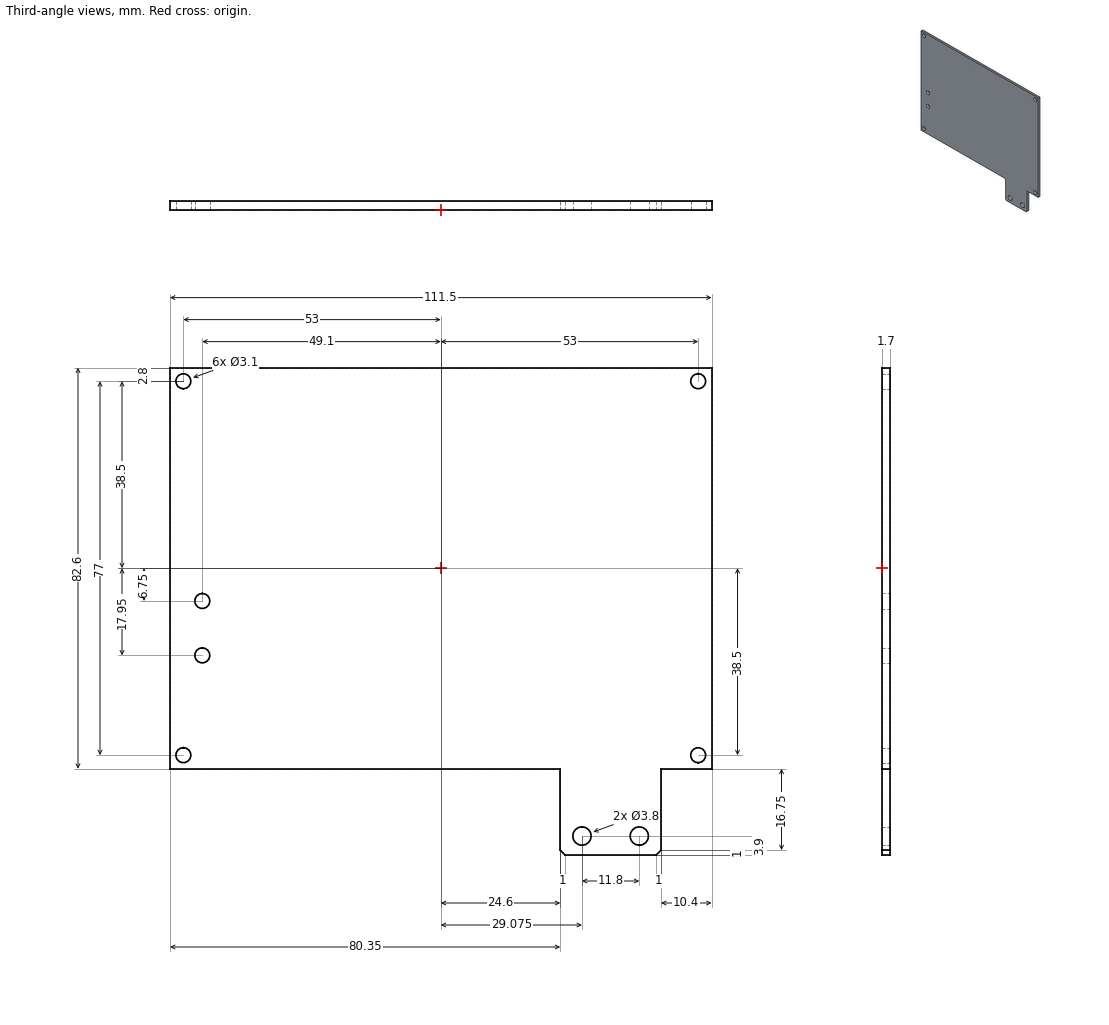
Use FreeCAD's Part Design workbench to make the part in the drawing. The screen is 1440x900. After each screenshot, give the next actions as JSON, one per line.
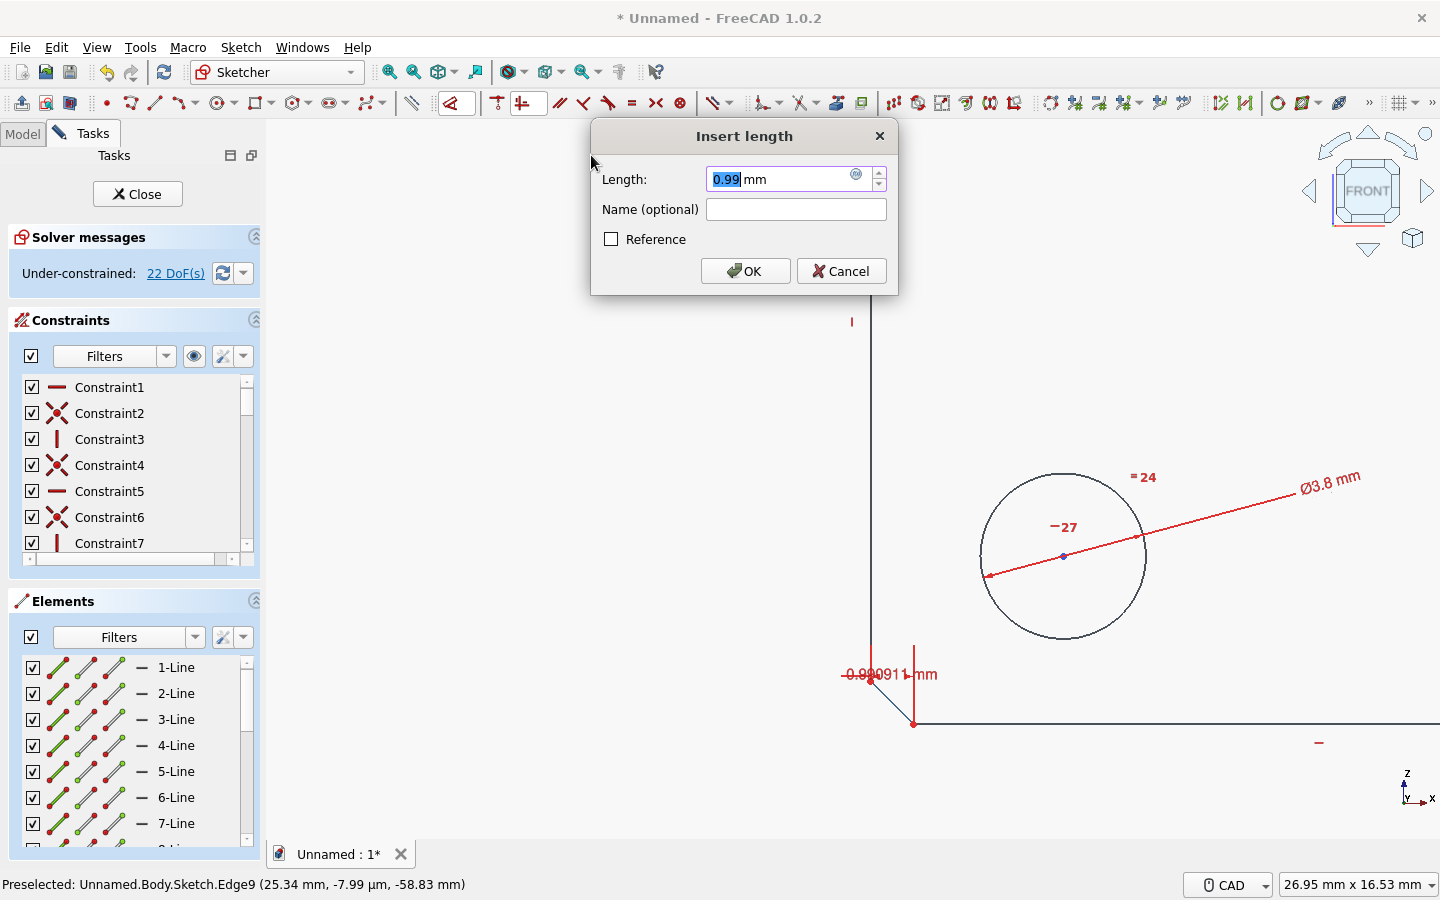
{"action": "type", "text": "1"}
{"action": "key", "text": "Return"}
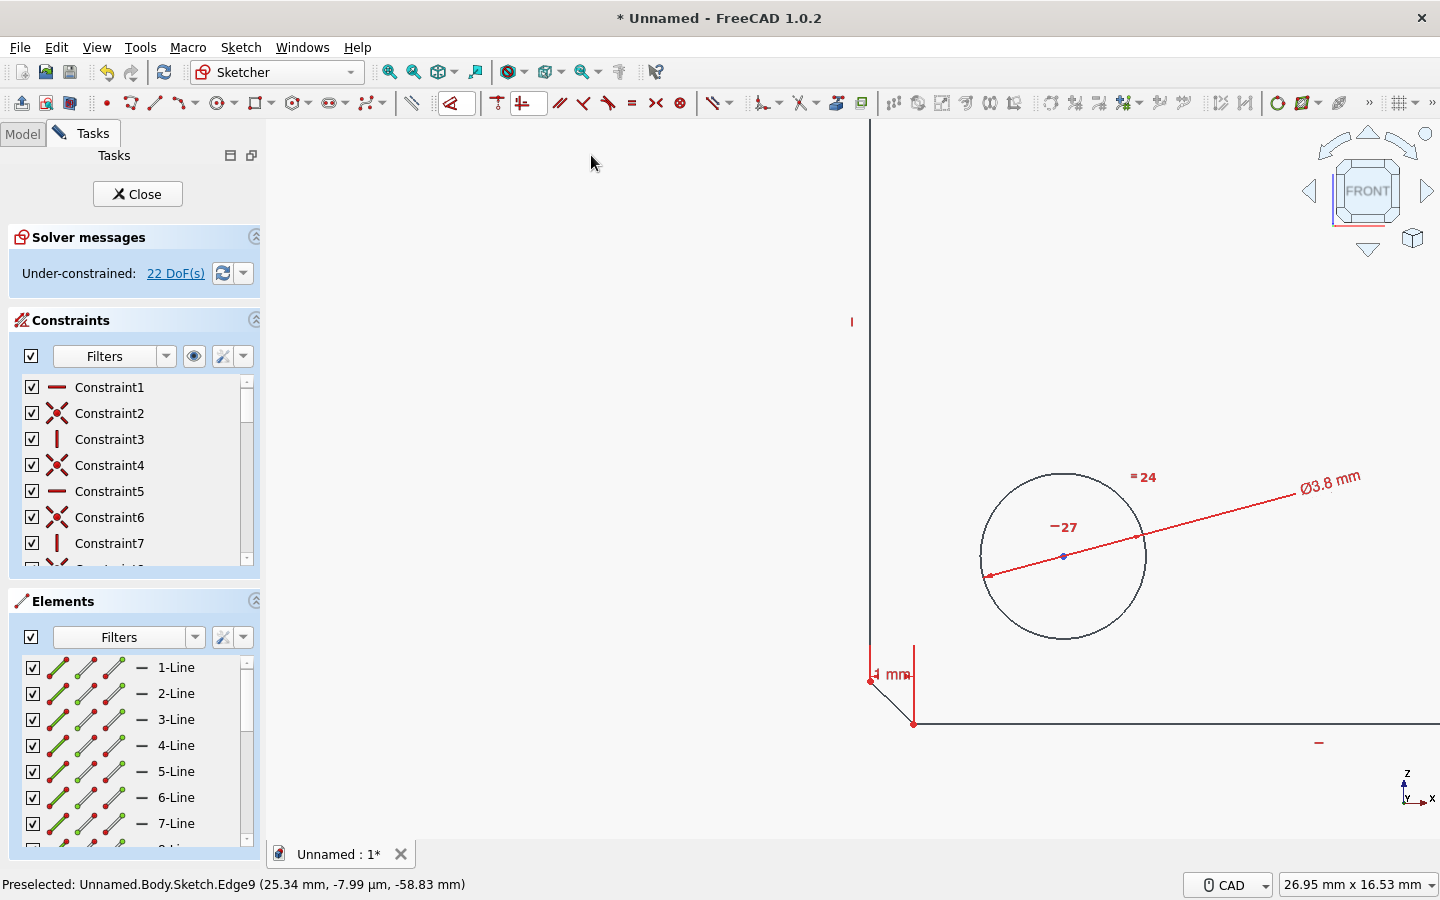
{"action": "left_click", "coordinate": [901, 712]}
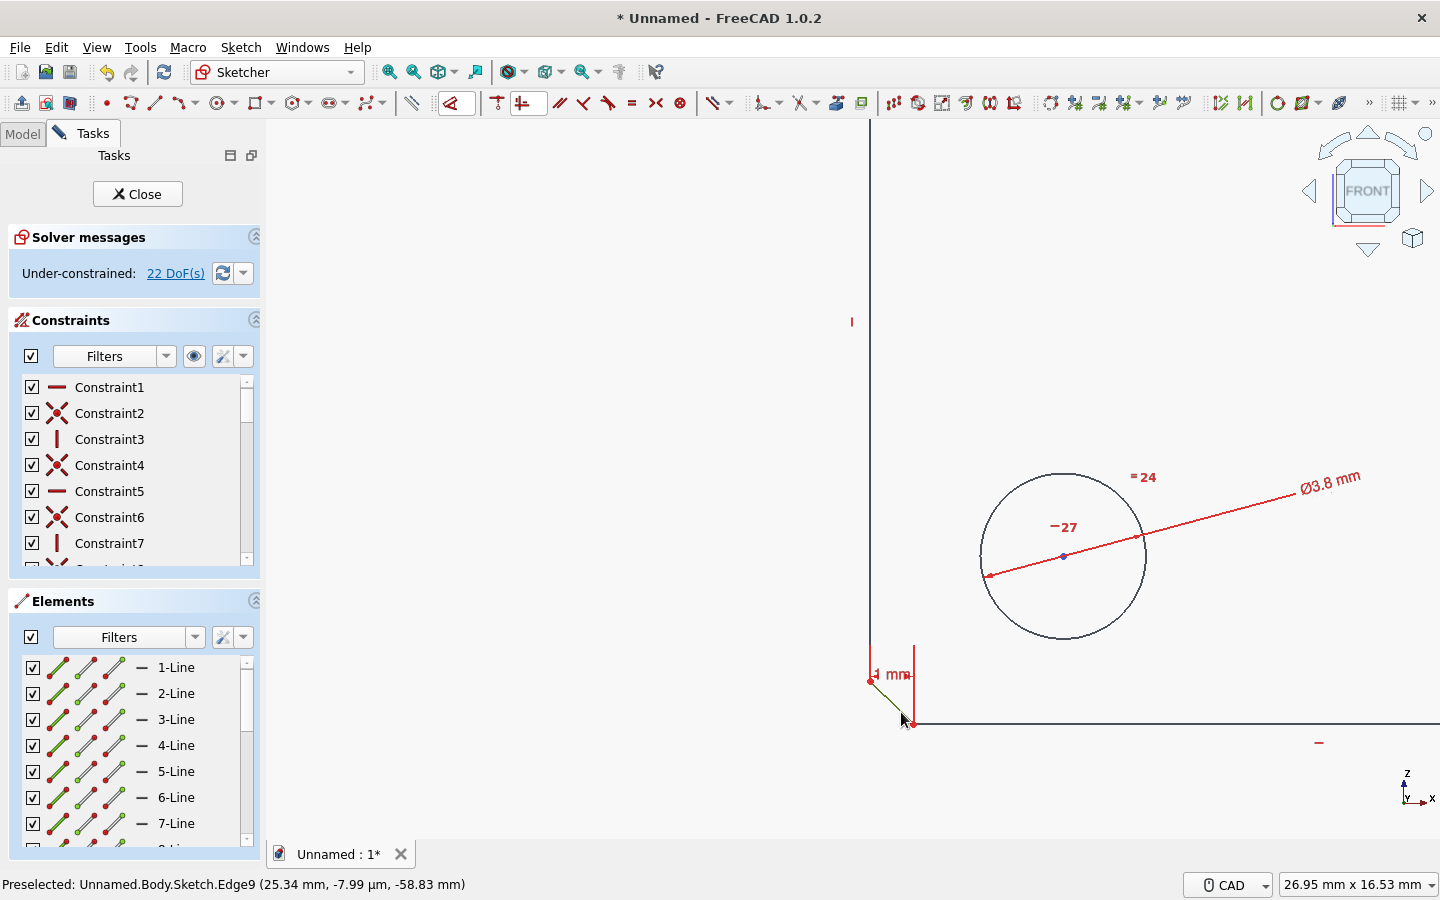
{"action": "left_click", "coordinate": [470, 104]}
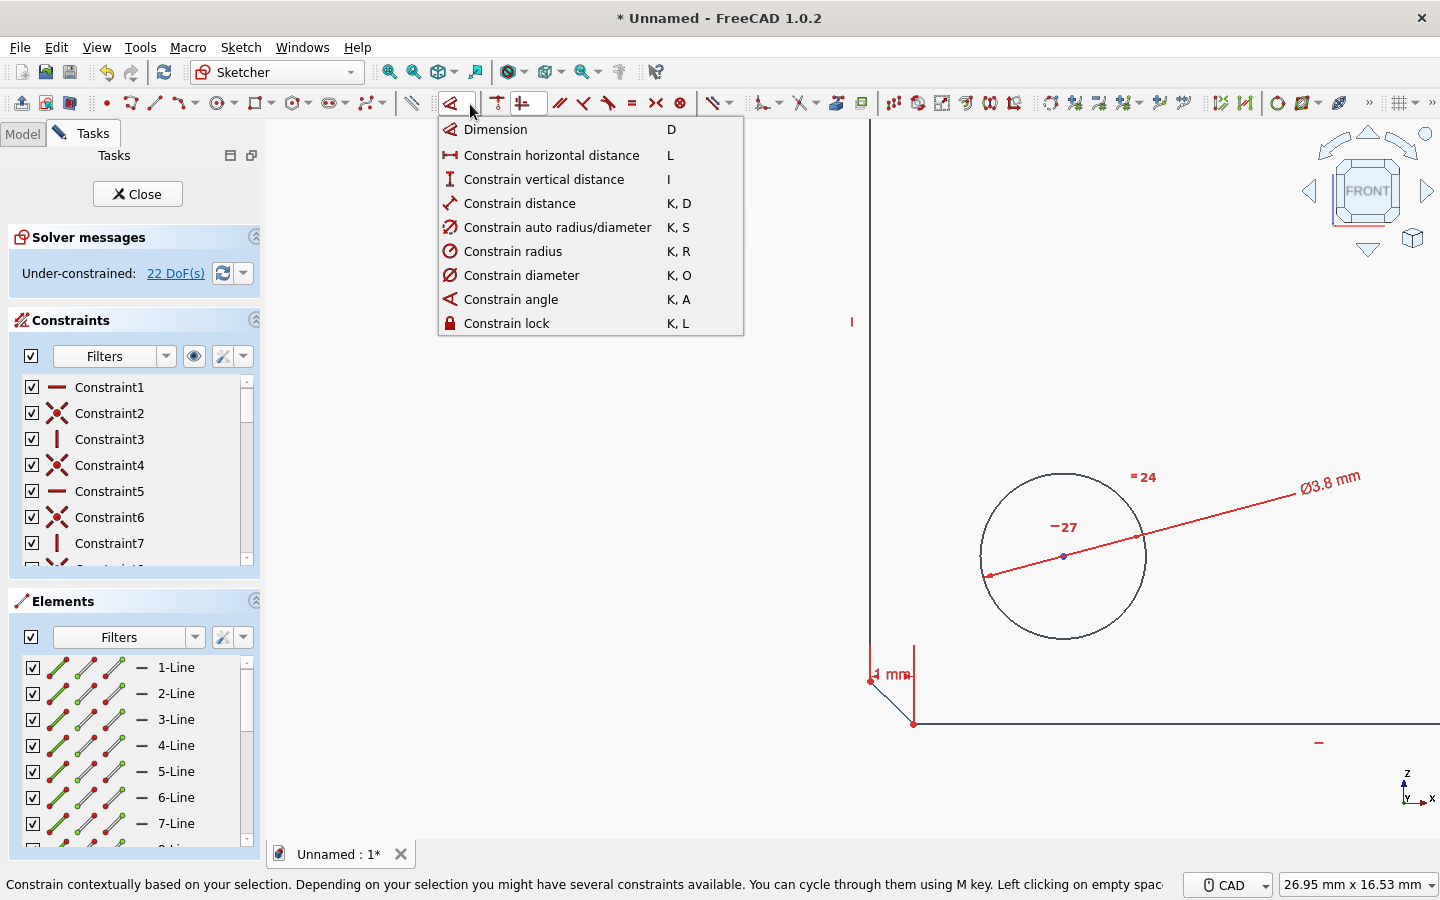
{"action": "left_click", "coordinate": [591, 179]}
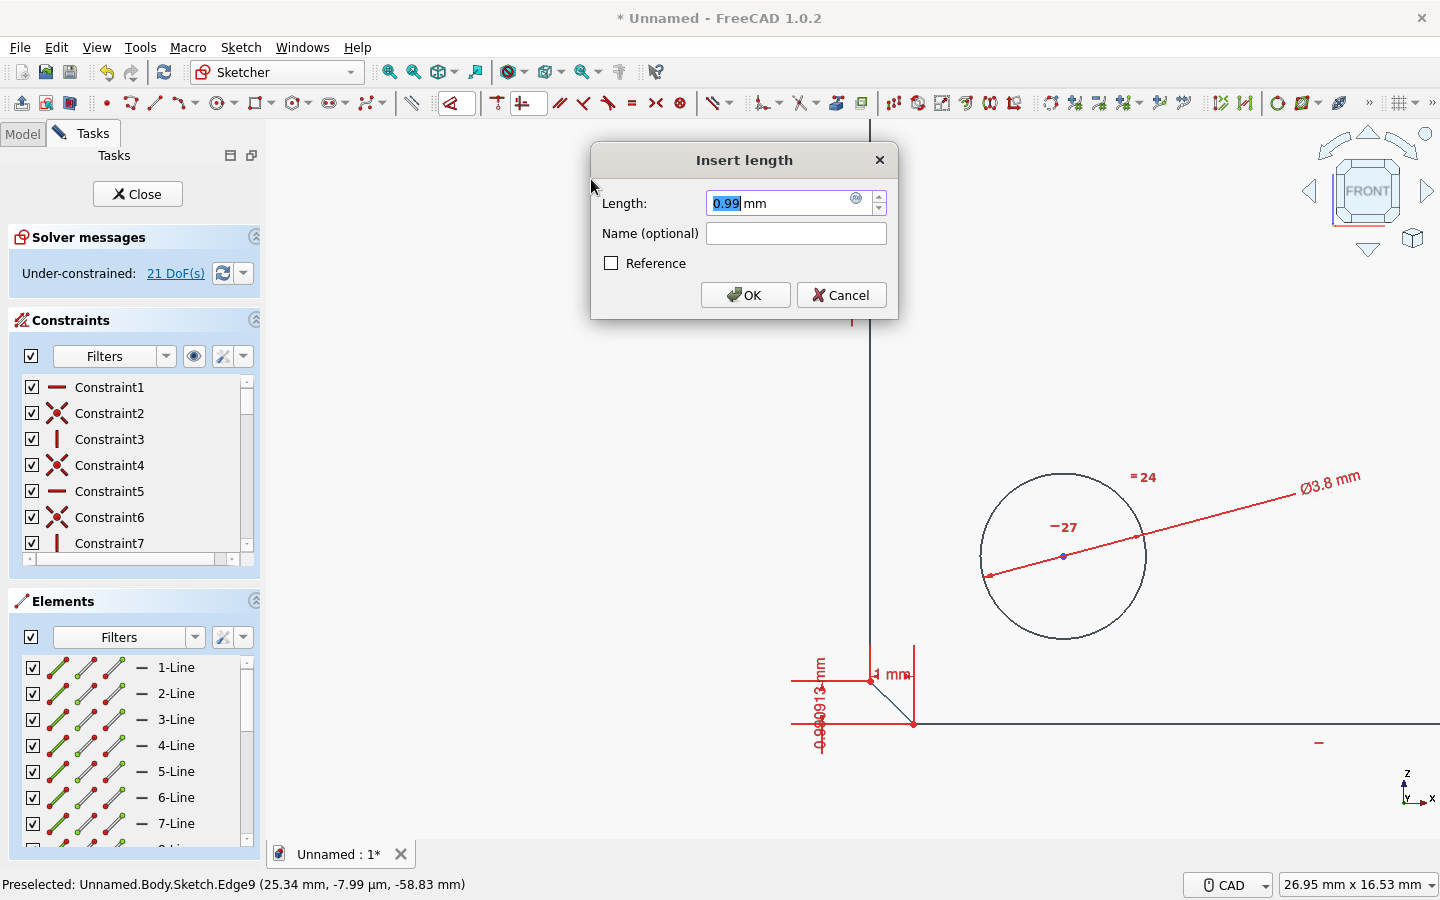
{"action": "type", "text": "1"}
{"action": "key", "text": "Return"}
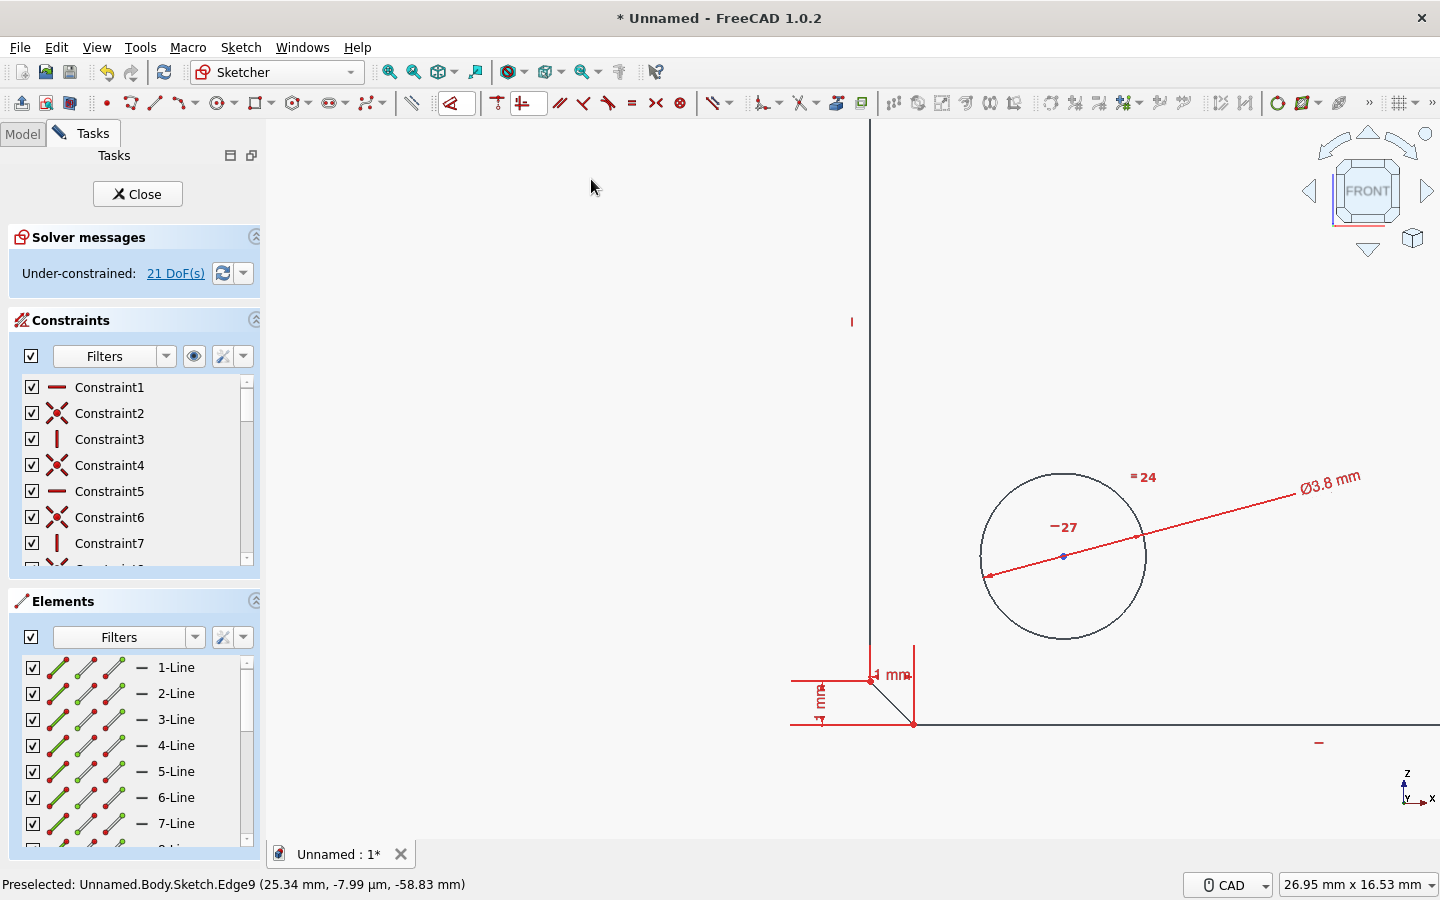
{"action": "scroll", "coordinate": [907, 721], "scroll_direction": "down", "scroll_amount": 11}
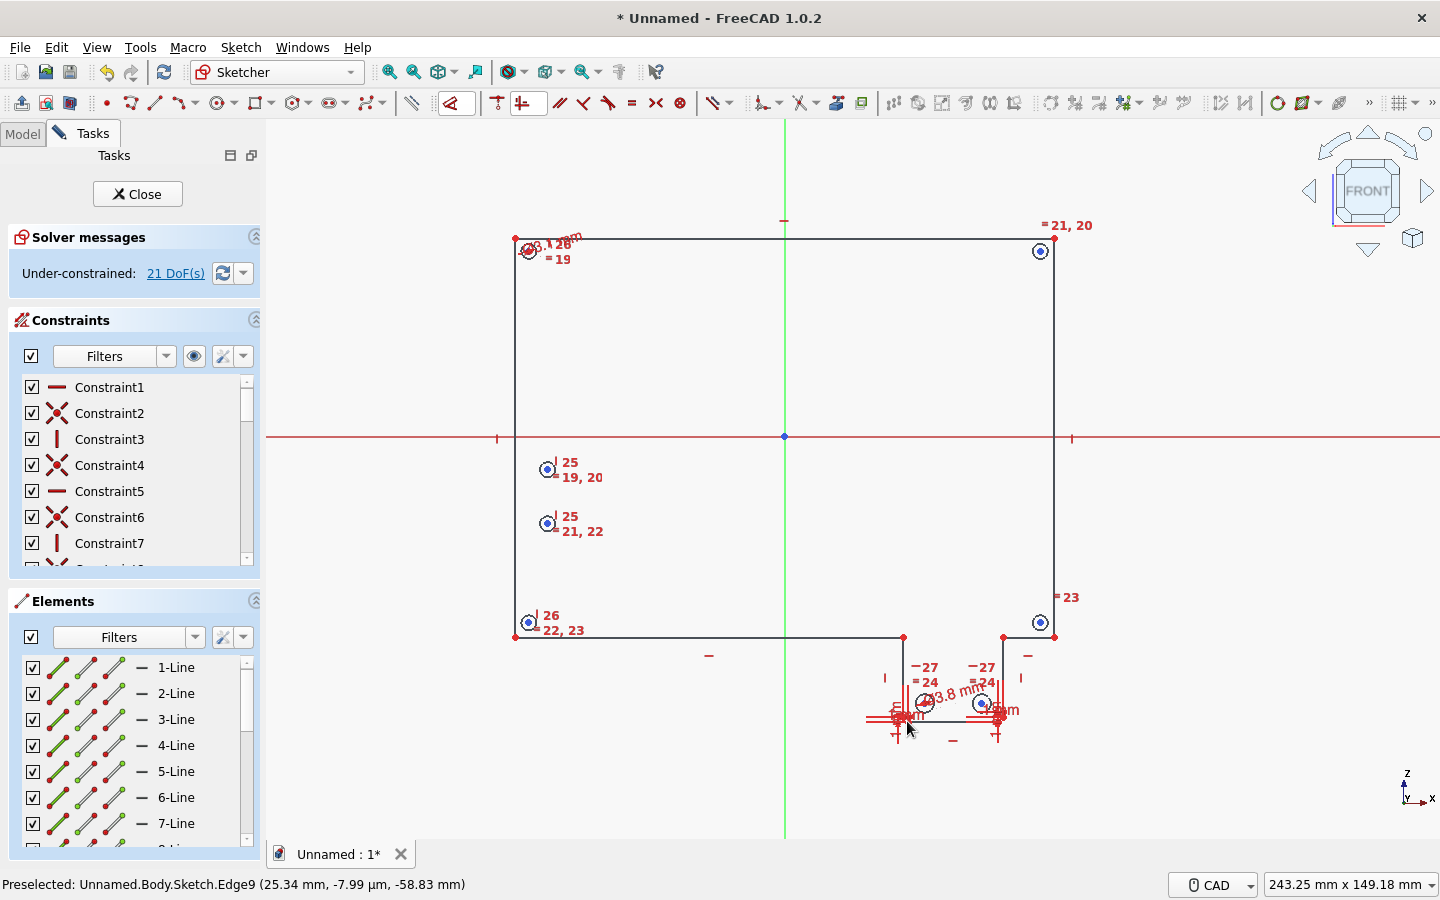
{"action": "left_click", "coordinate": [529, 251]}